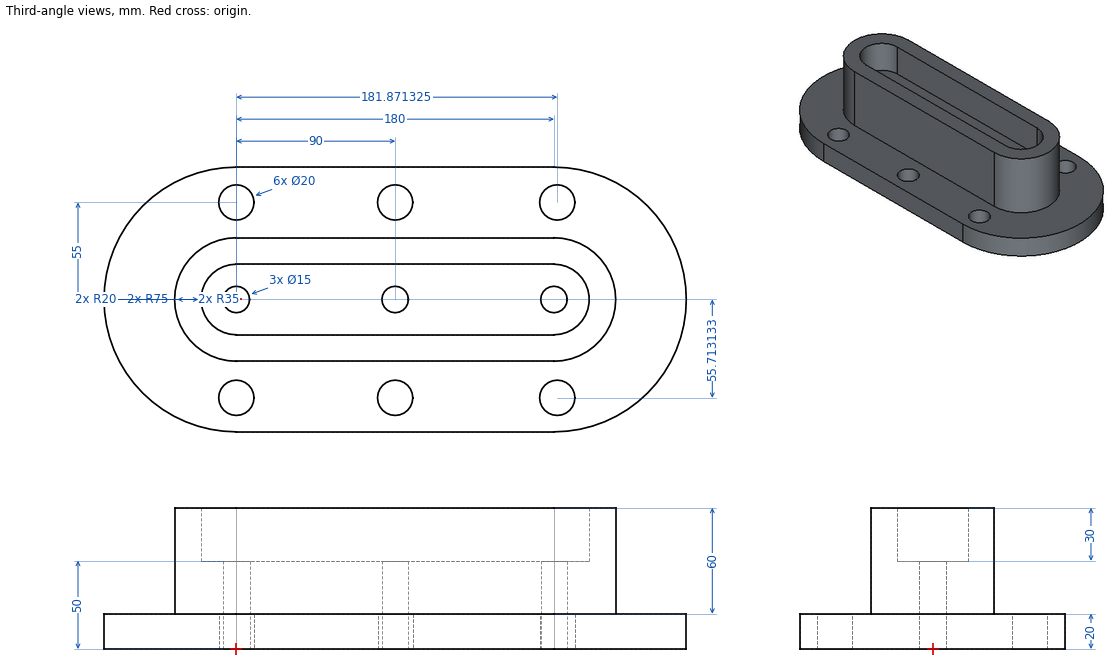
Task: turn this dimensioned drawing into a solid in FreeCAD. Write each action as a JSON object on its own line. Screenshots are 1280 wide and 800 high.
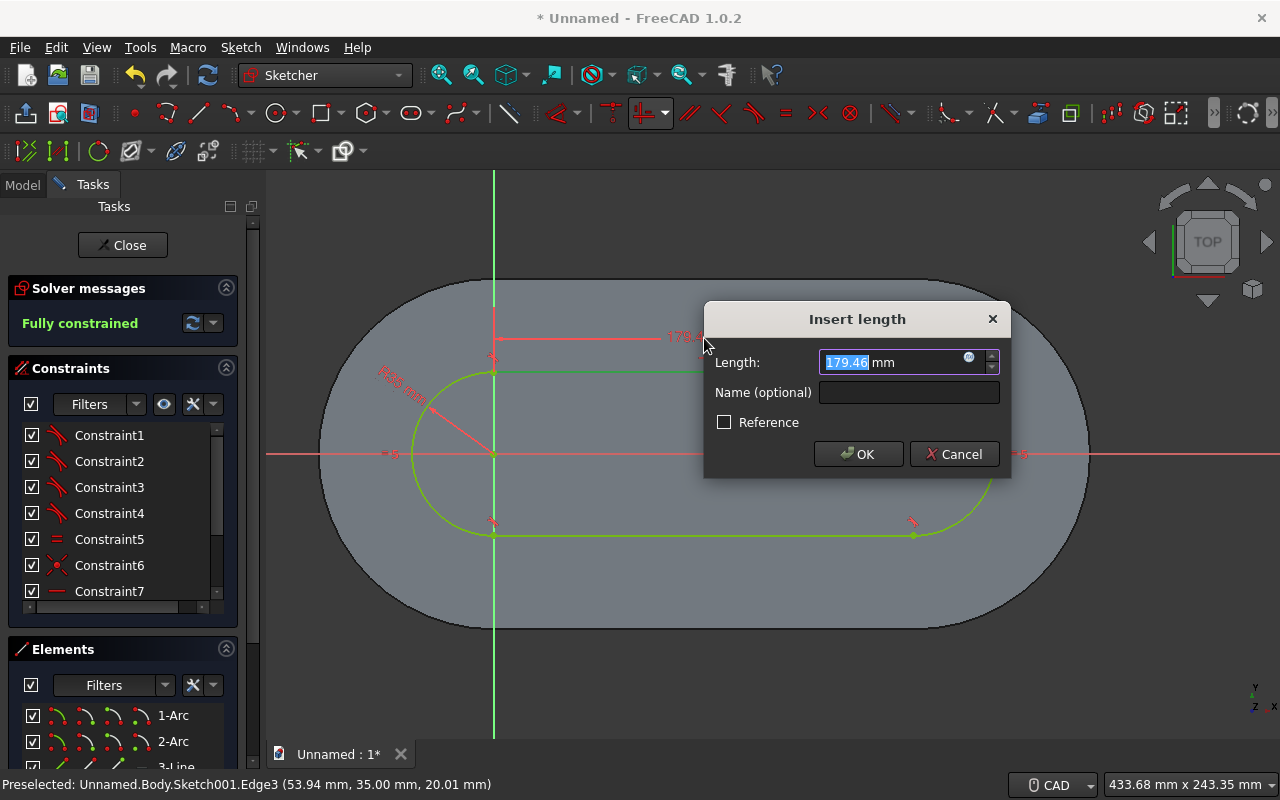
{"action": "type", "text": "180"}
{"action": "key", "text": "Return"}
{"action": "key", "text": "Escape"}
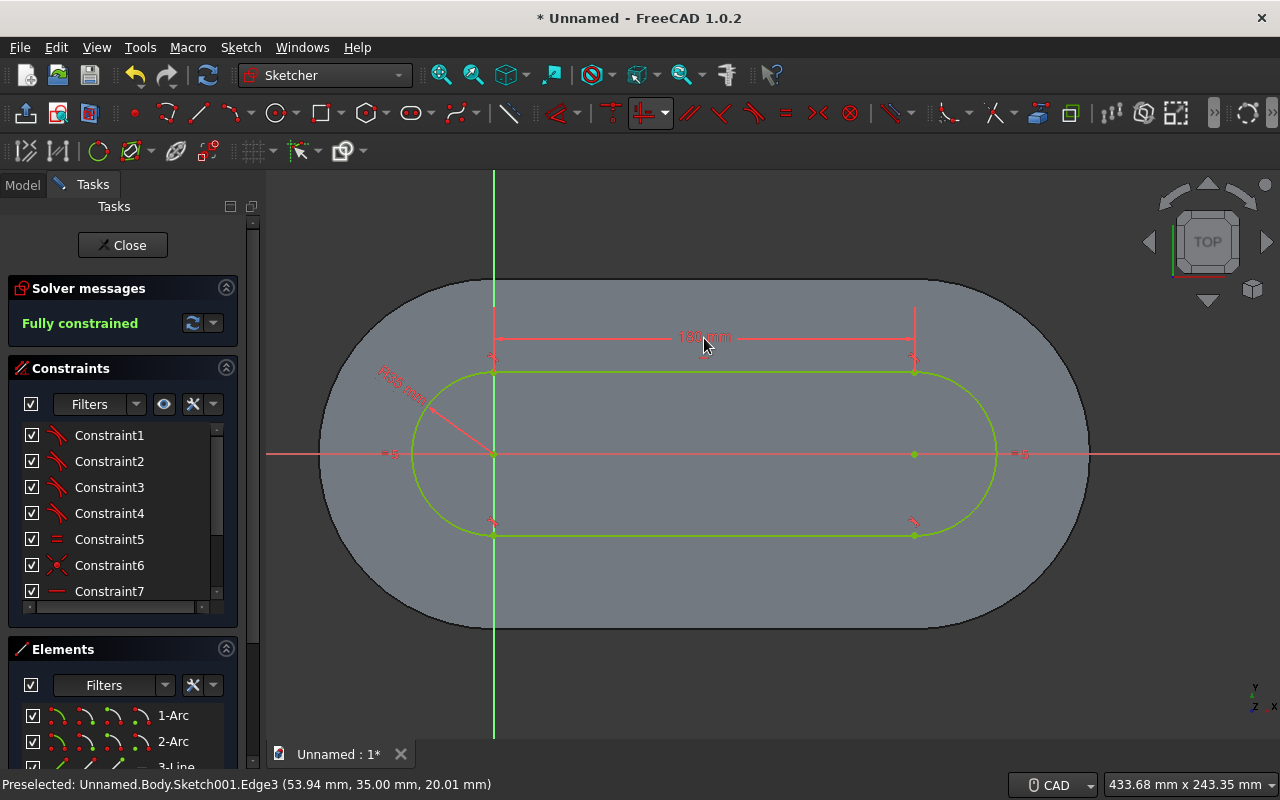
{"action": "left_click", "coordinate": [123, 245]}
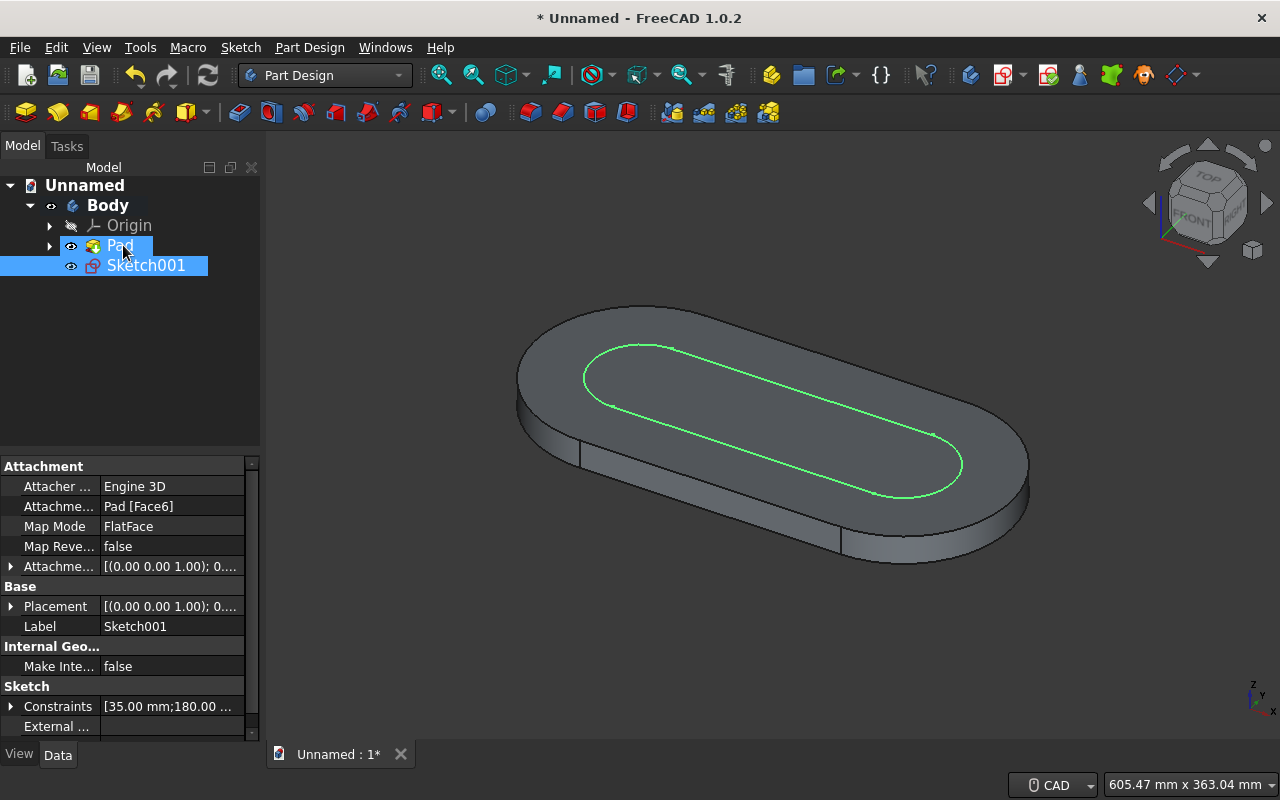
{"action": "left_click", "coordinate": [26, 112]}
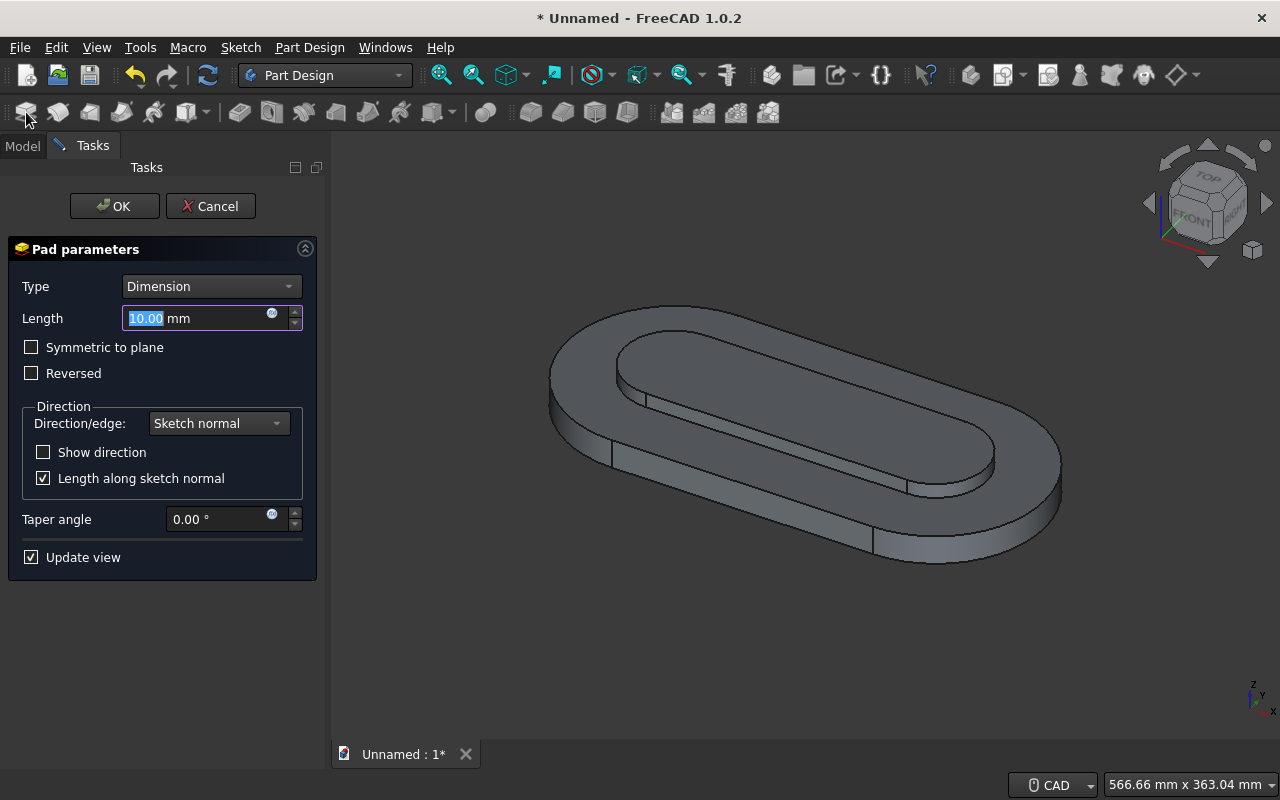
{"action": "type", "text": "60"}
{"action": "key", "text": "Tab"}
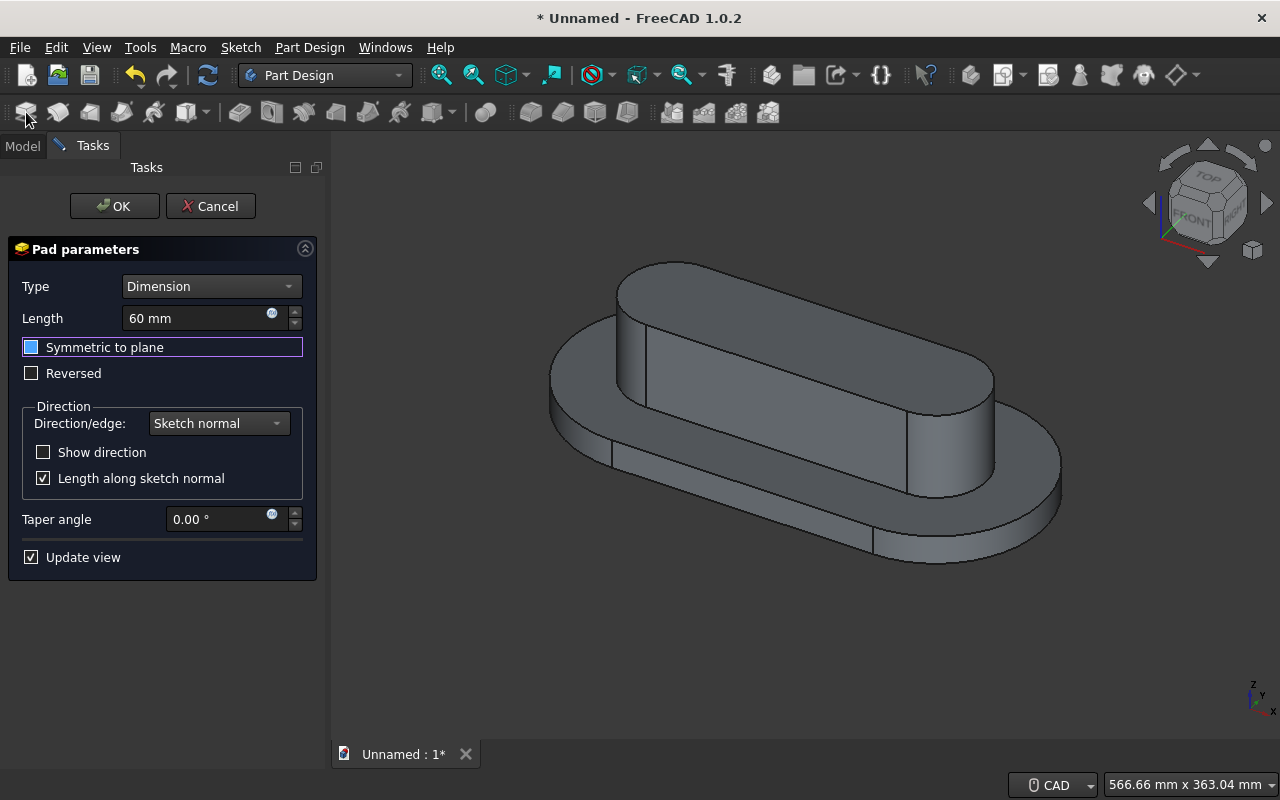
{"action": "left_click", "coordinate": [115, 206]}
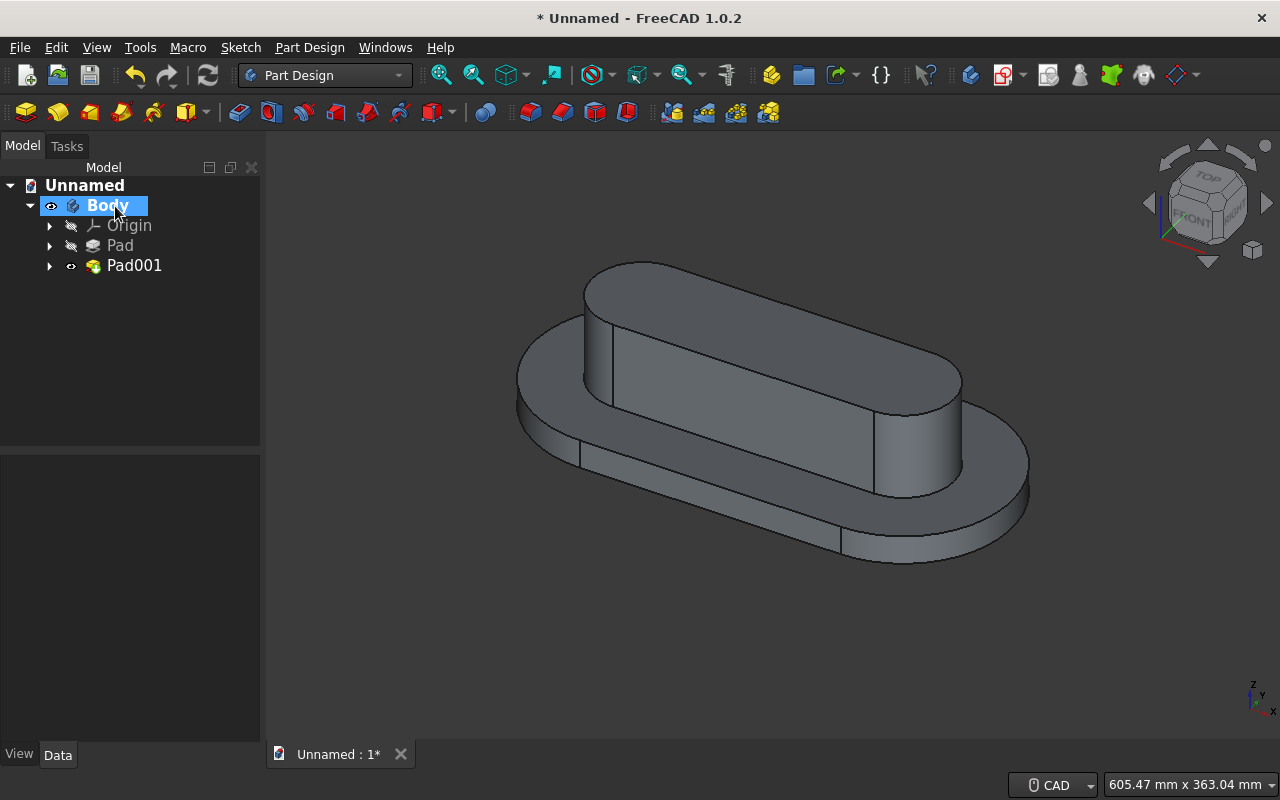
{"action": "left_click", "coordinate": [877, 372]}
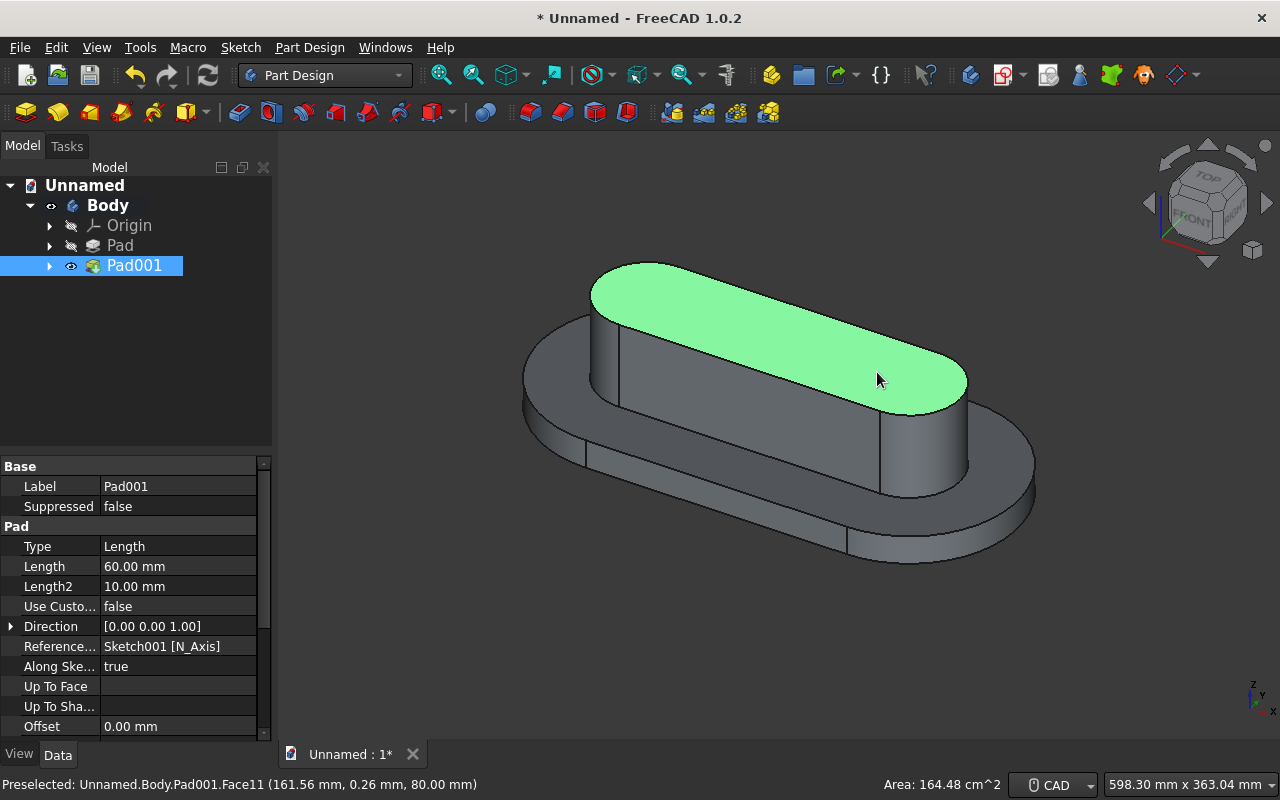
{"action": "left_click", "coordinate": [1004, 76]}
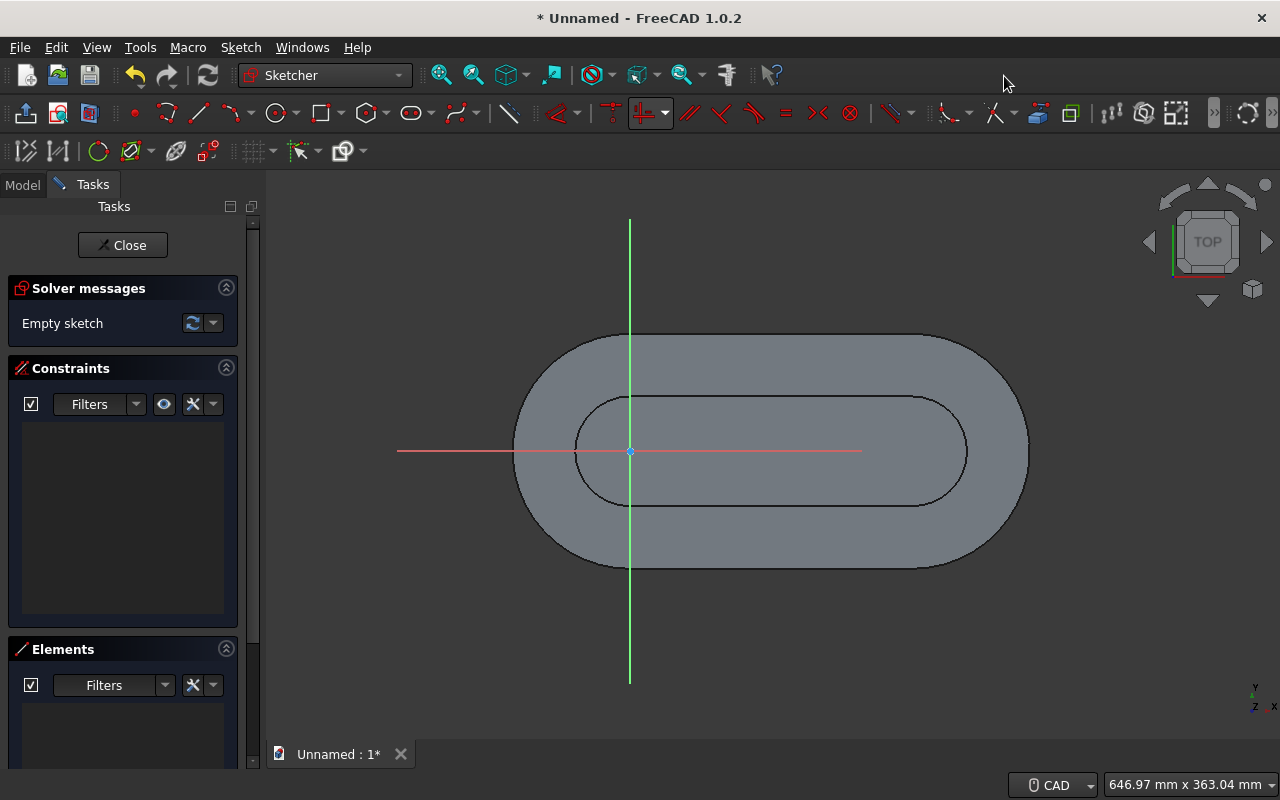
{"action": "scroll", "coordinate": [852, 447], "scroll_direction": "up", "scroll_amount": 3}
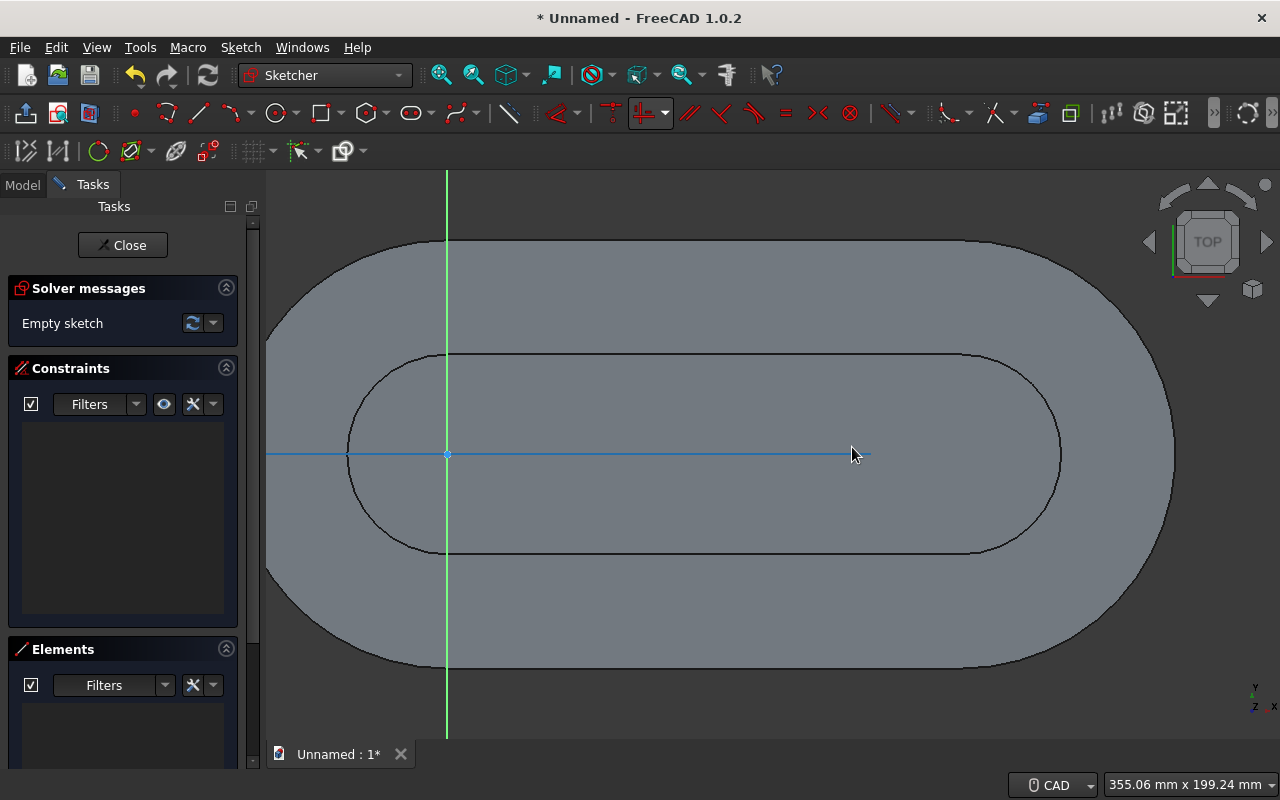
{"action": "left_click", "coordinate": [412, 114]}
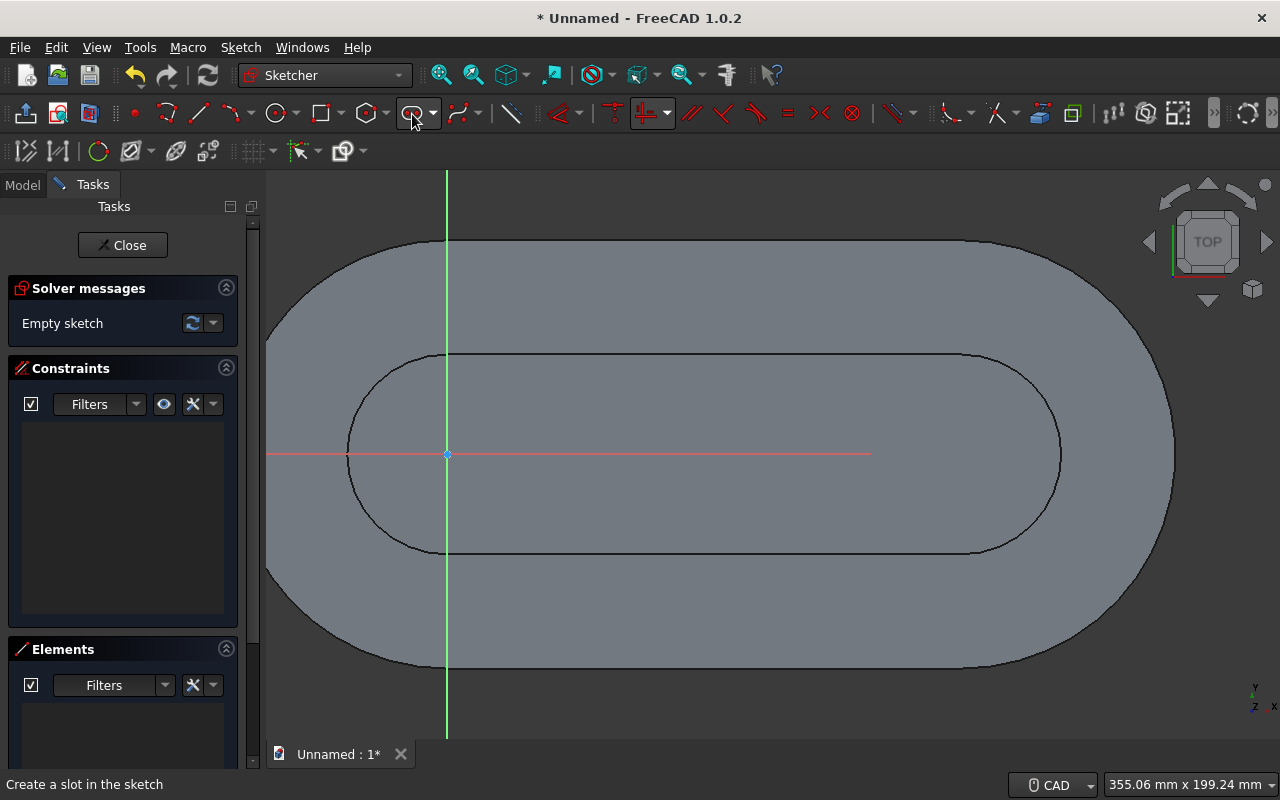
{"action": "left_click", "coordinate": [447, 454]}